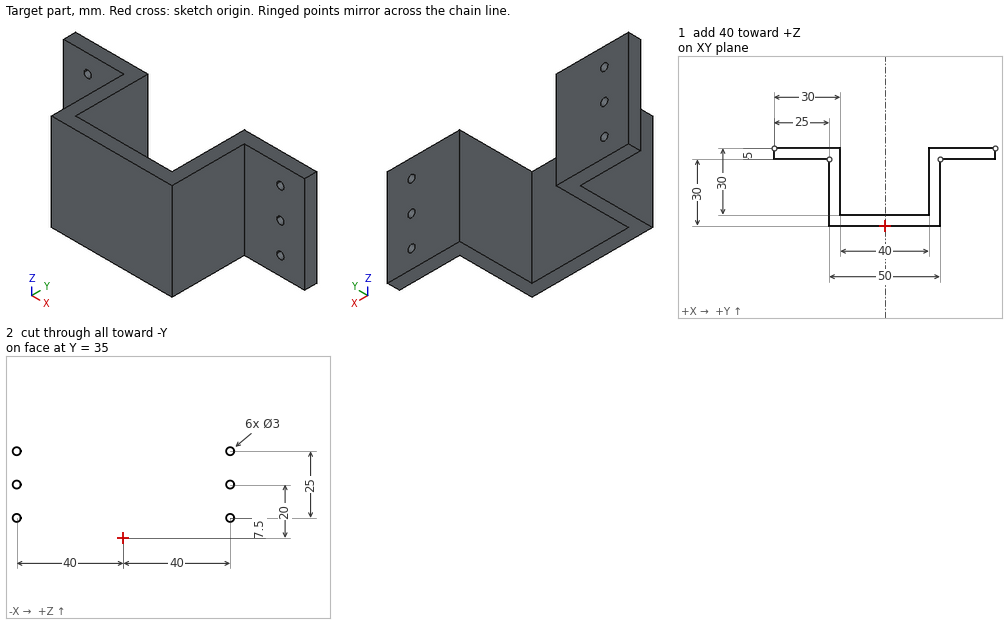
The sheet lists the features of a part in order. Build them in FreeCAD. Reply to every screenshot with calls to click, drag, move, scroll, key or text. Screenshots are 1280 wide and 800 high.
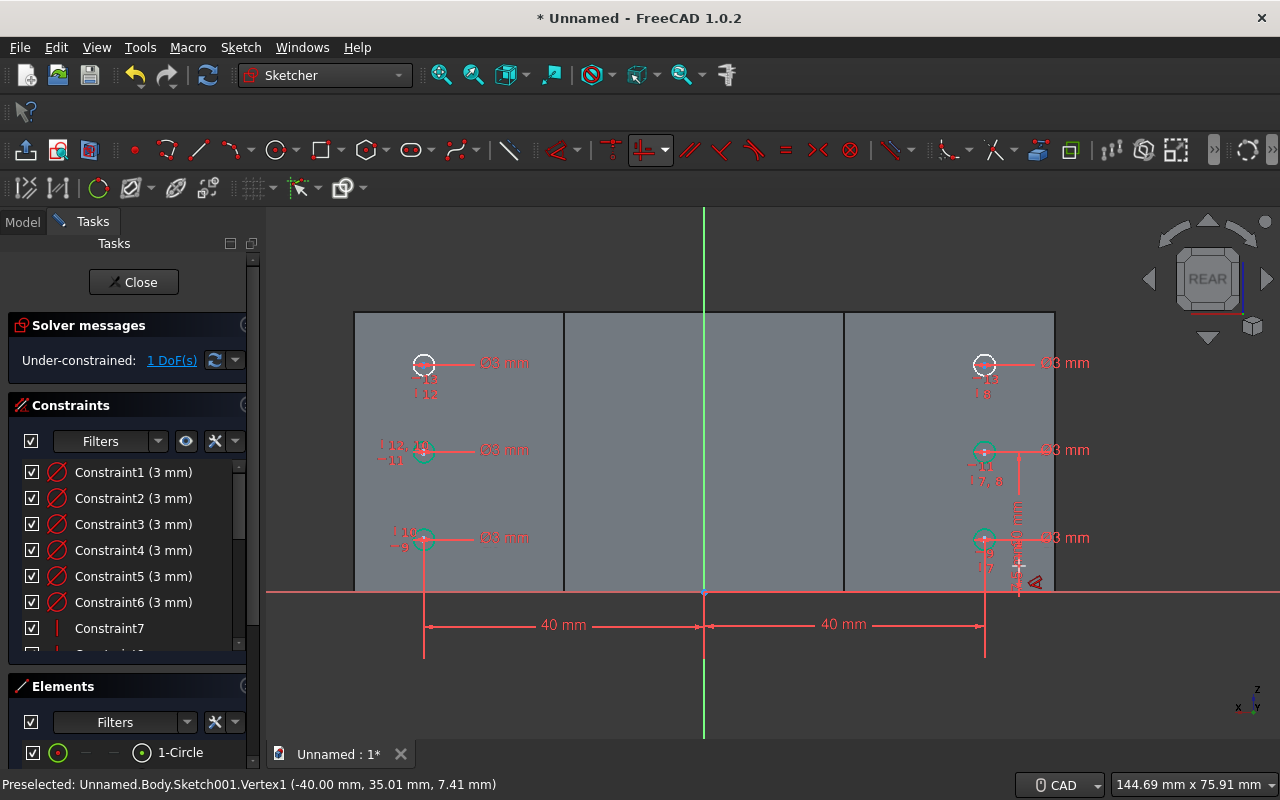
click(985, 540)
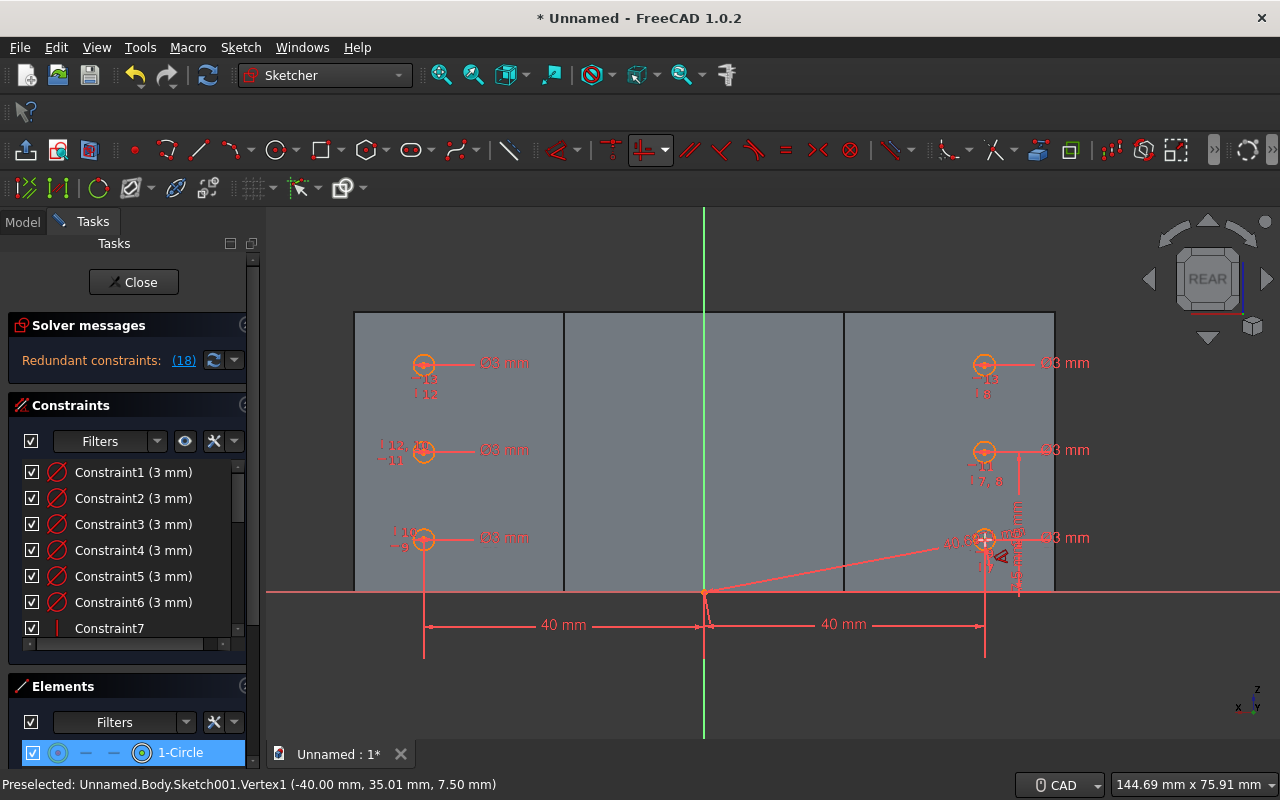
click(985, 365)
click(1019, 452)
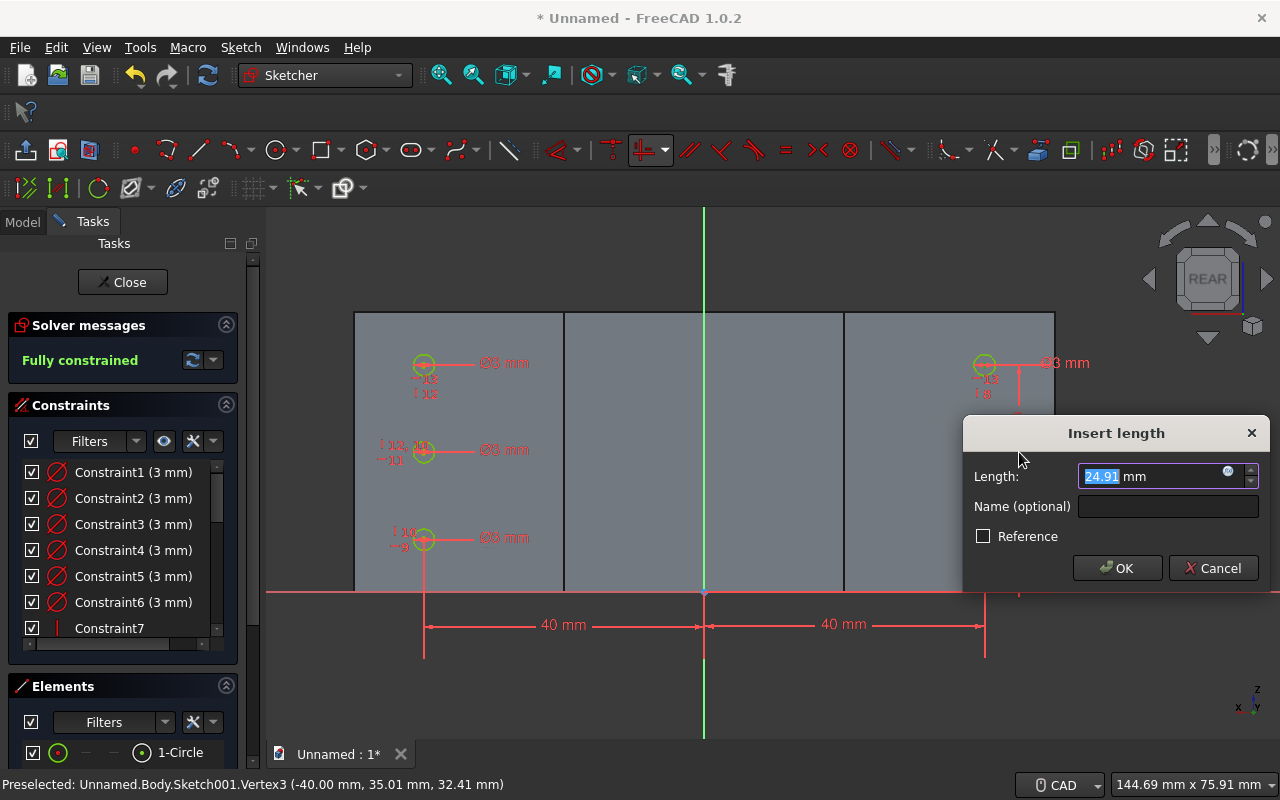
text(25)
key(Return)
key(Escape)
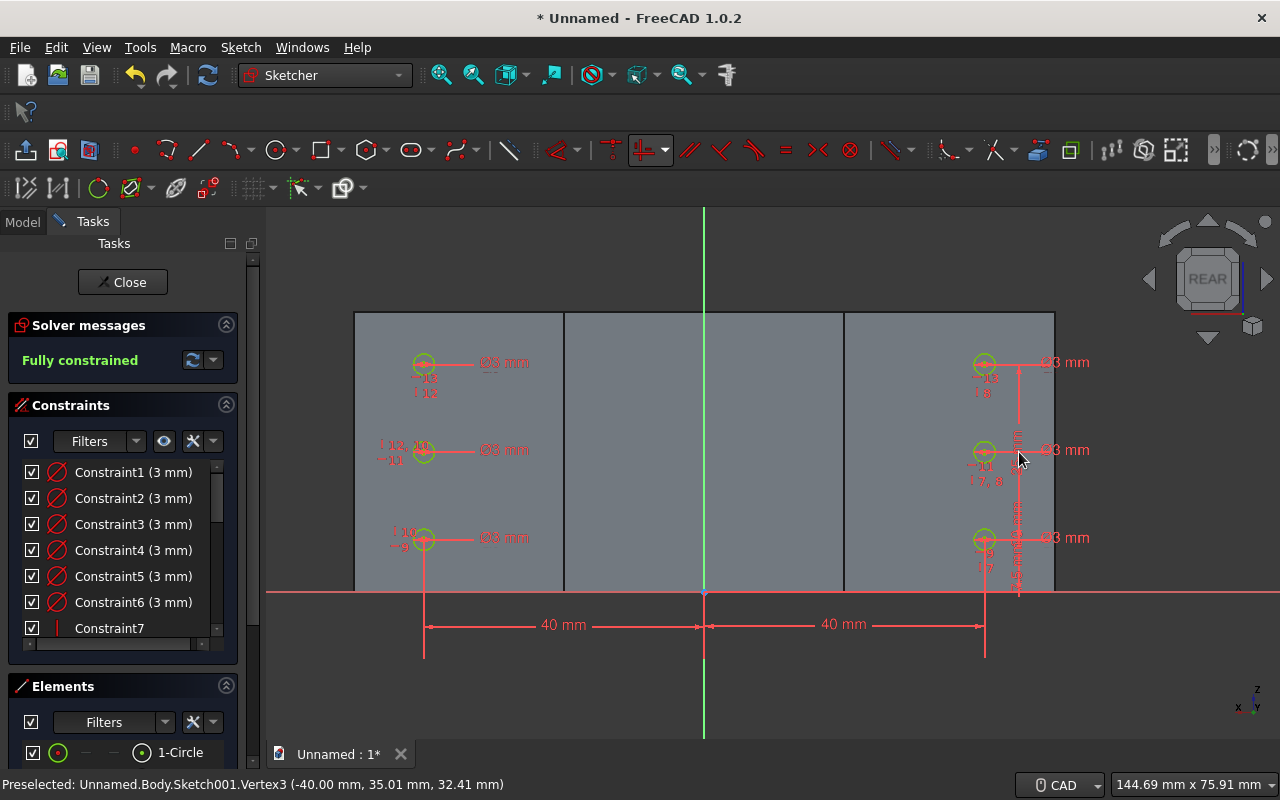
click(123, 282)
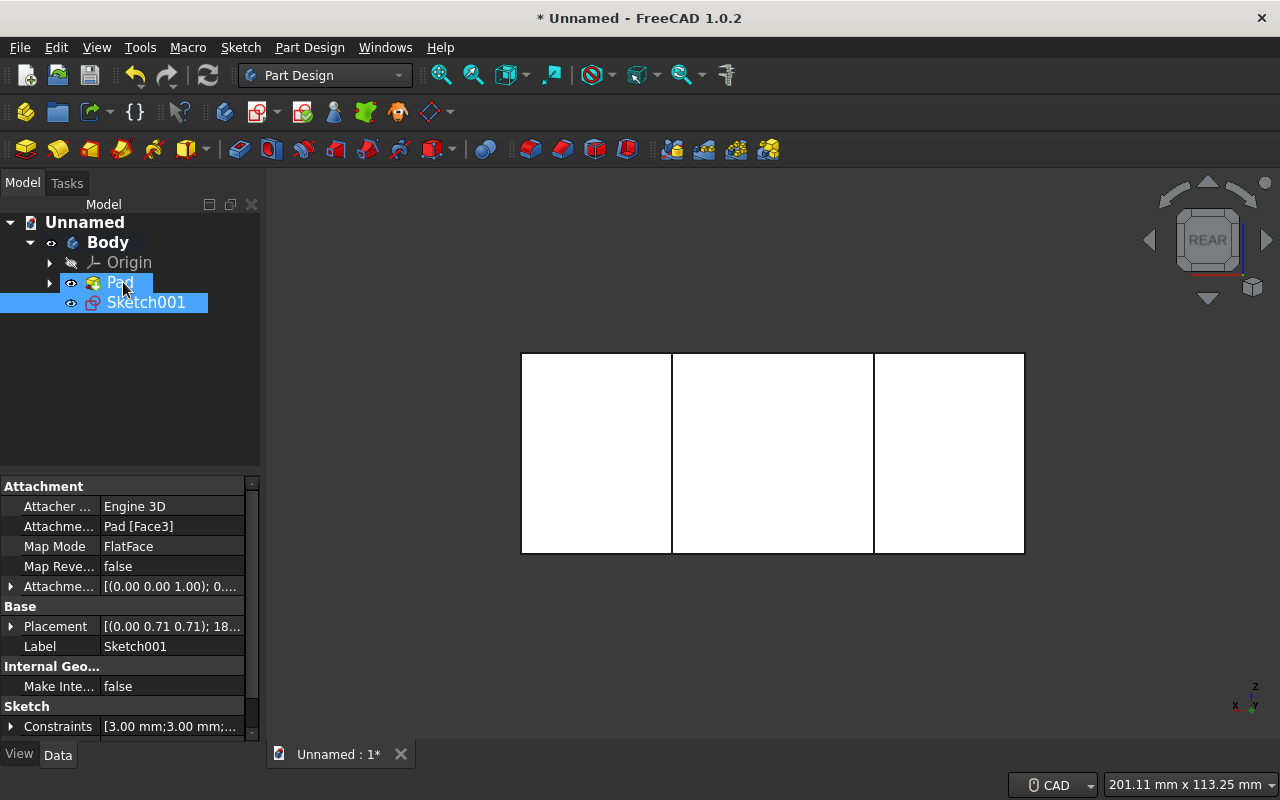
click(240, 150)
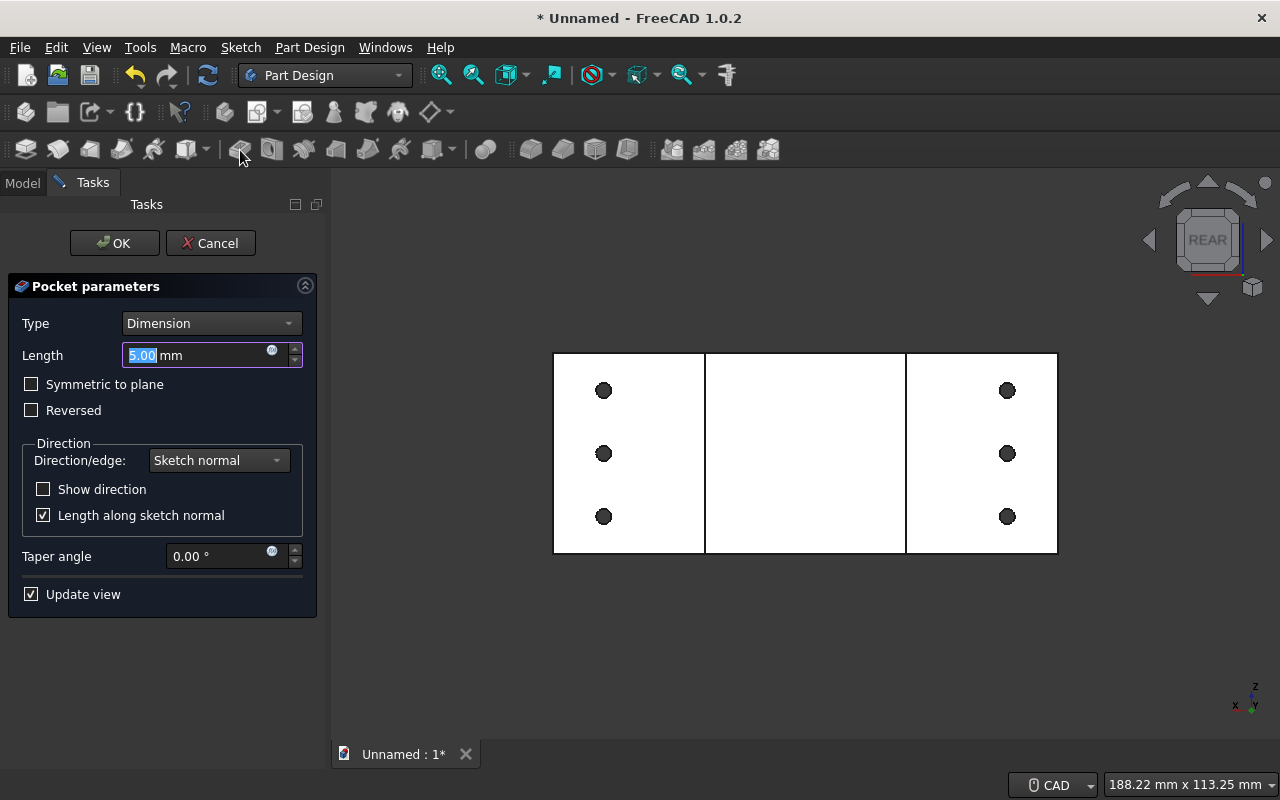
click(212, 324)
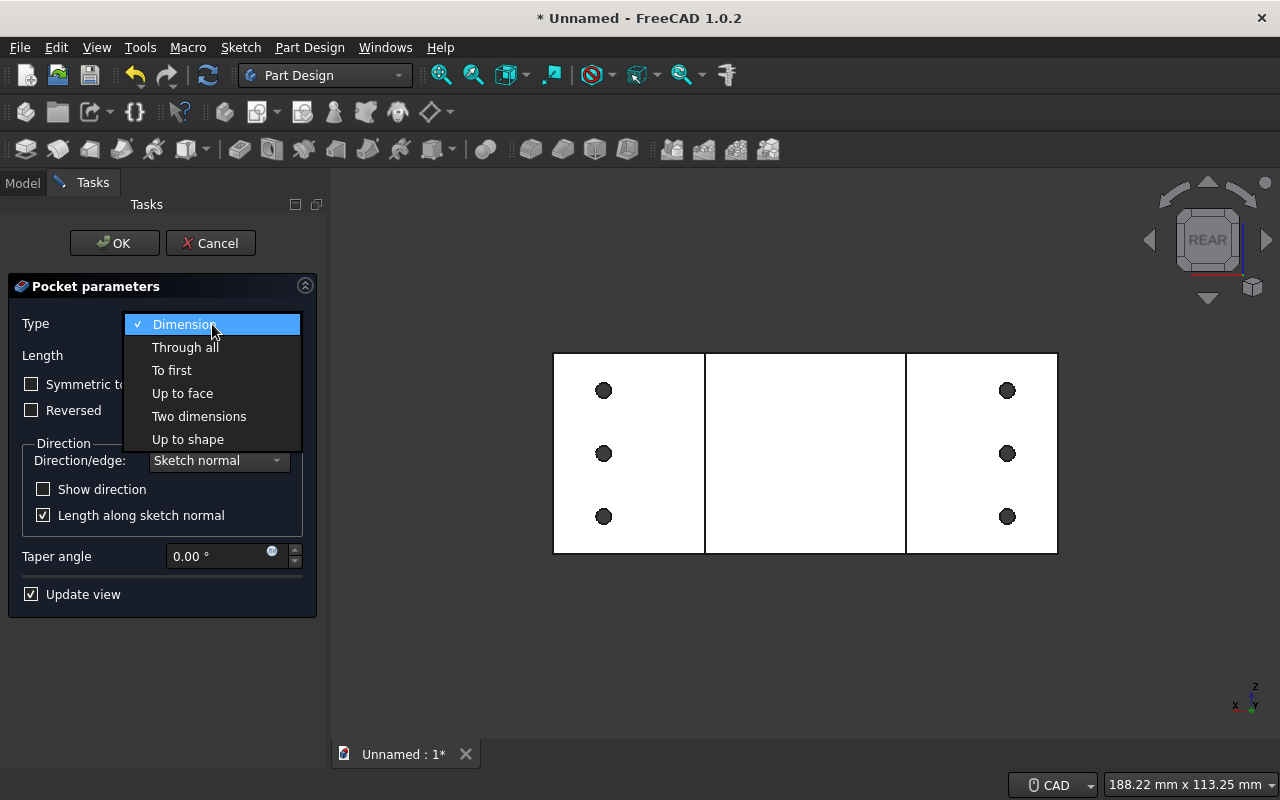
click(212, 348)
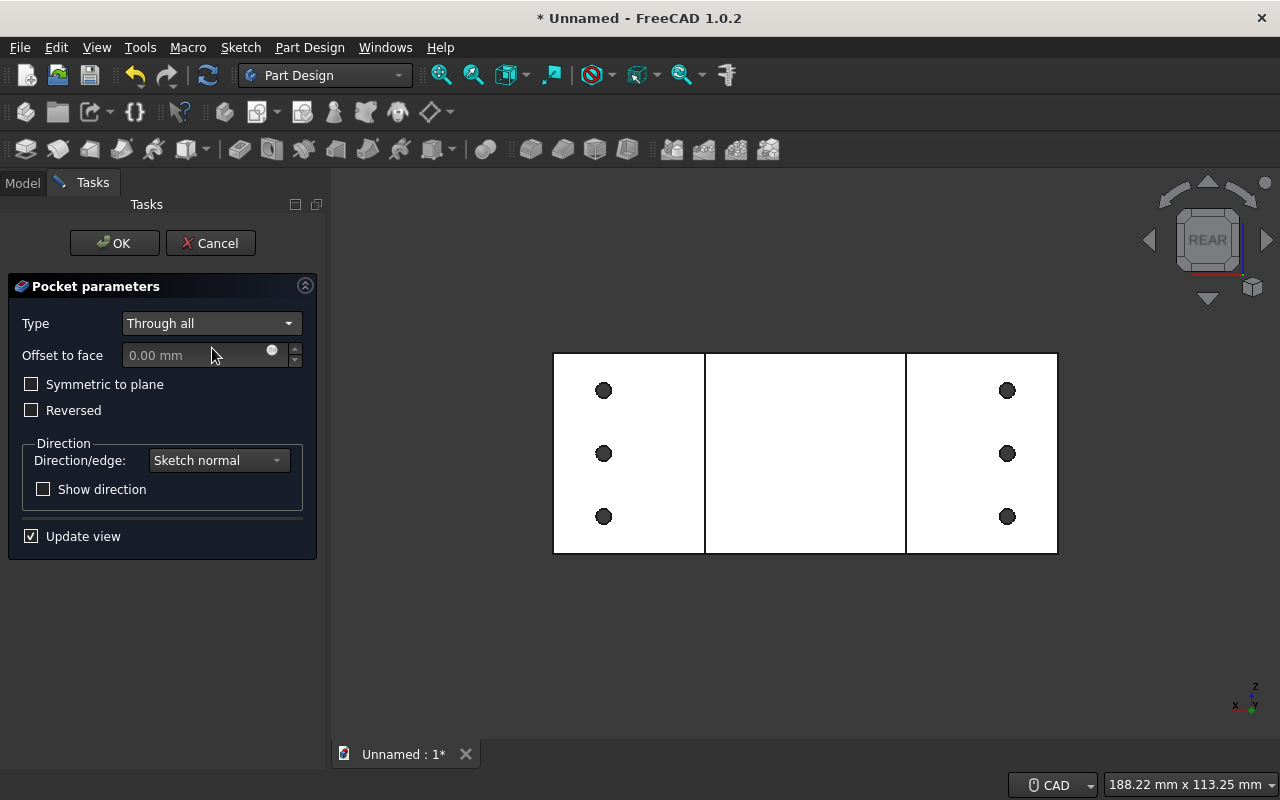
click(115, 243)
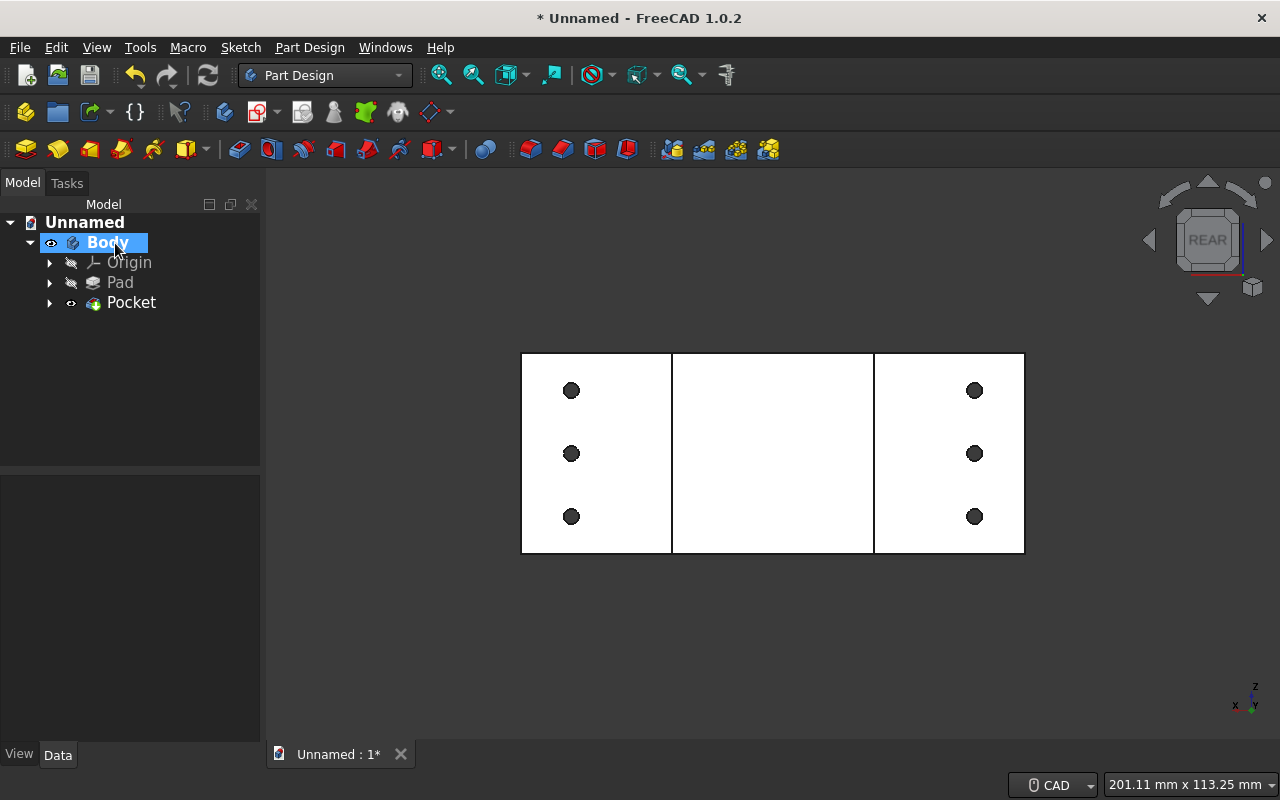
key(0)